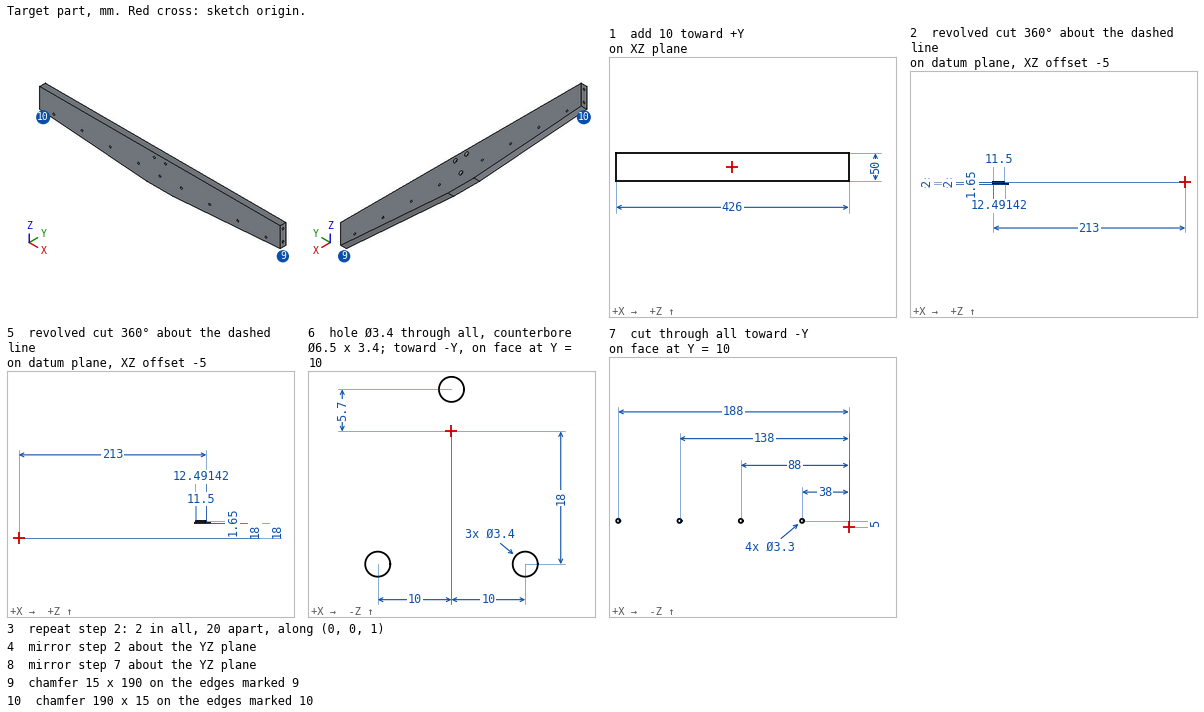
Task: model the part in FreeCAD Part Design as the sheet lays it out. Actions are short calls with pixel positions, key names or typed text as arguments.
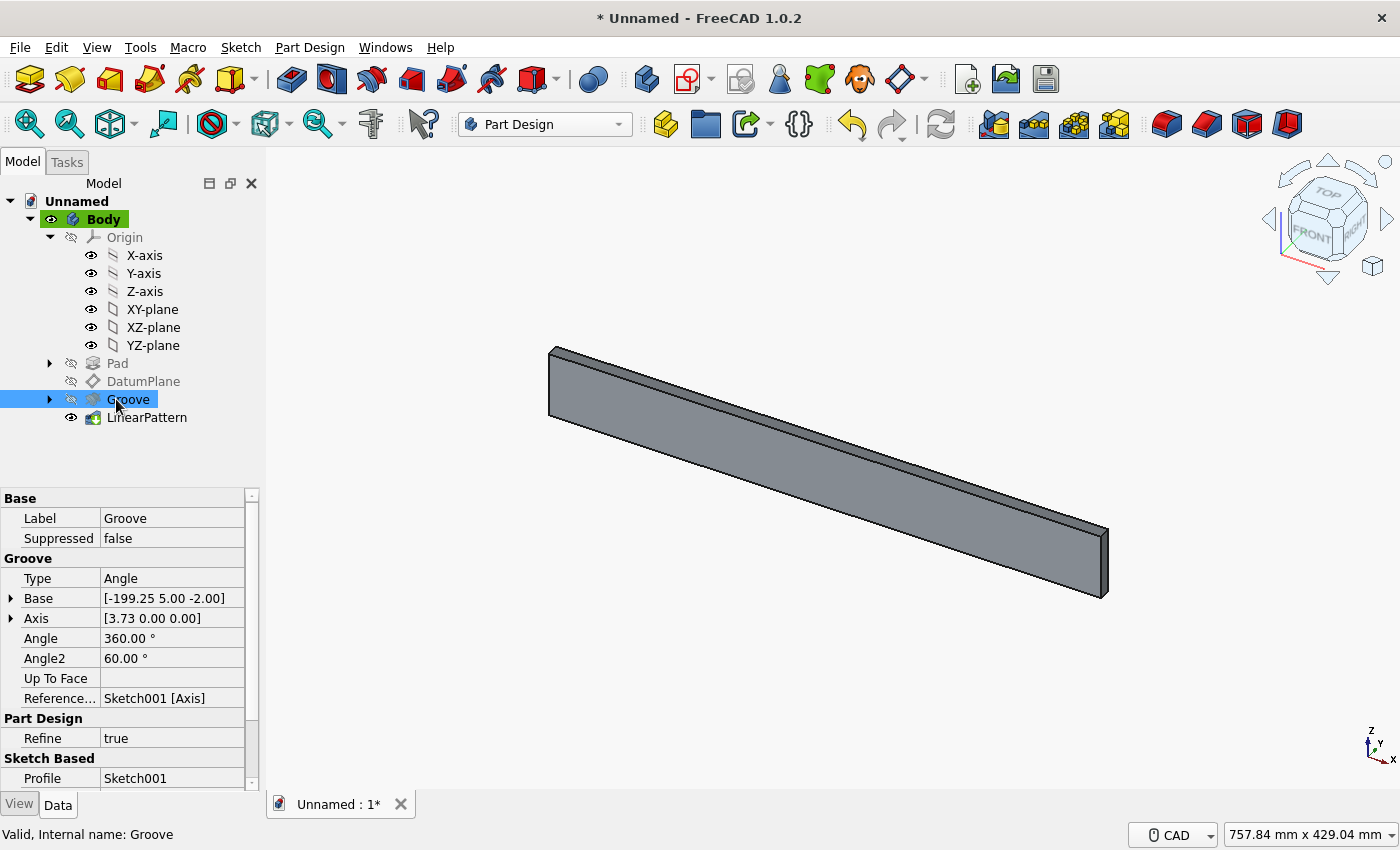
click(994, 124)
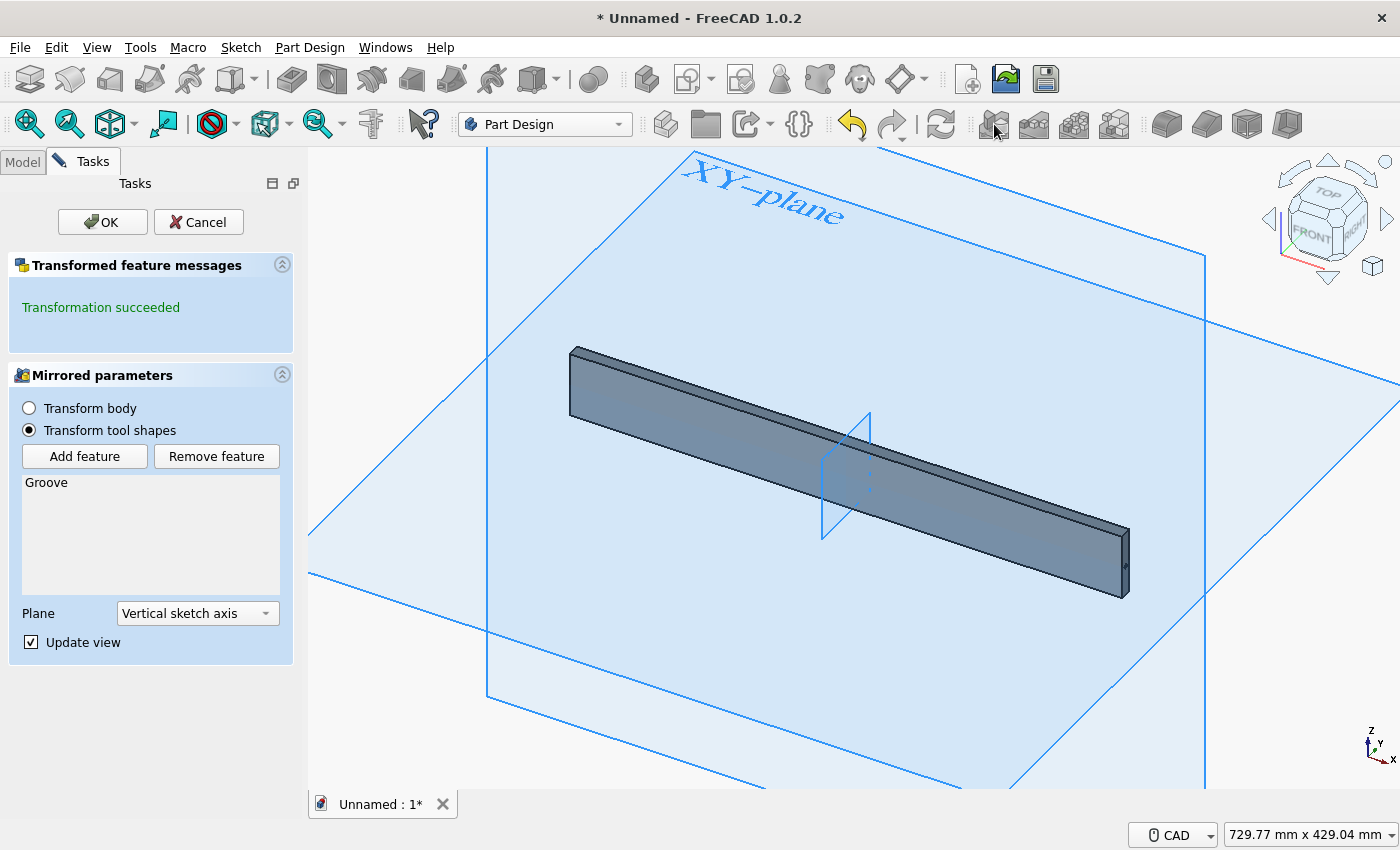
click(198, 614)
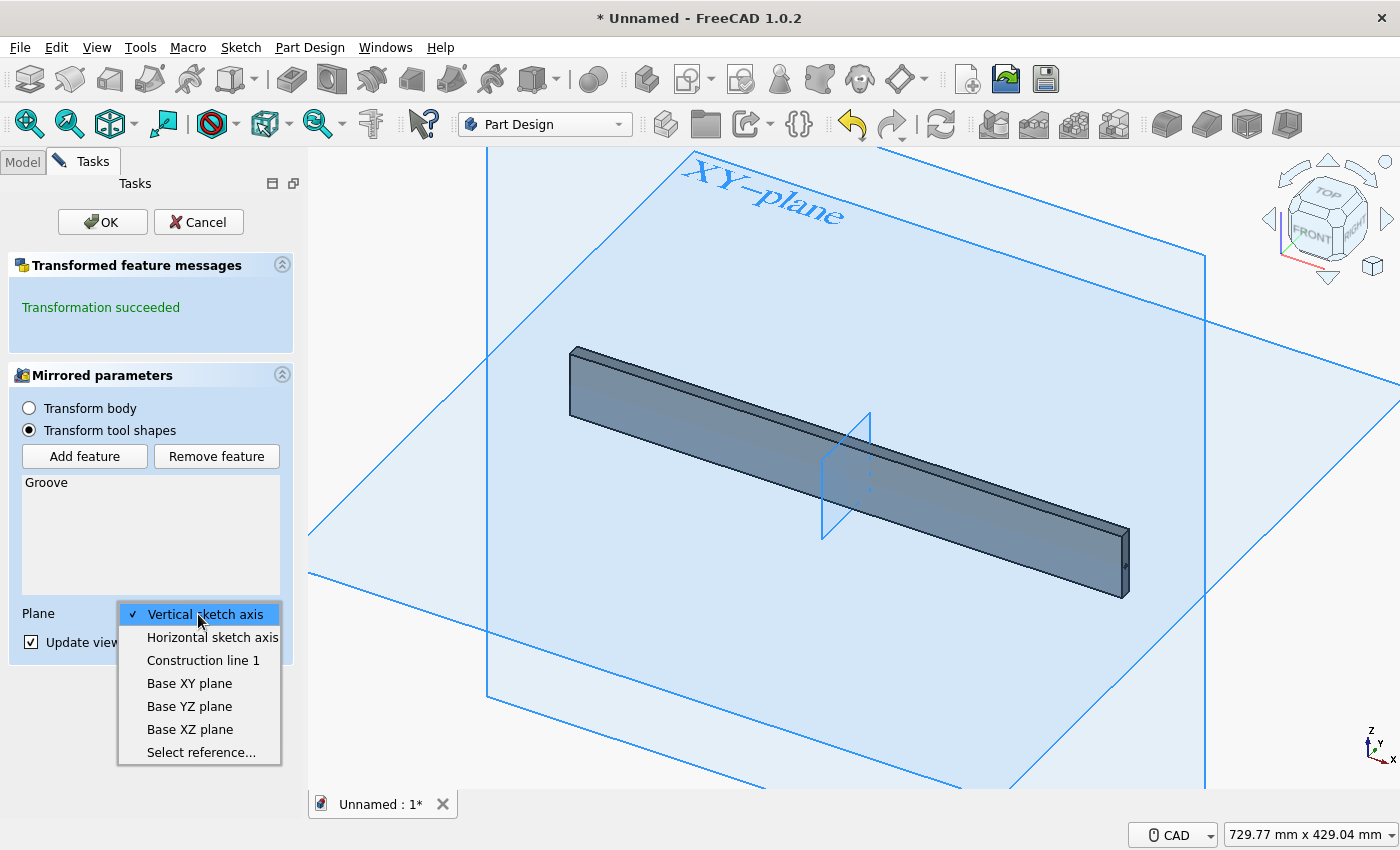
click(198, 706)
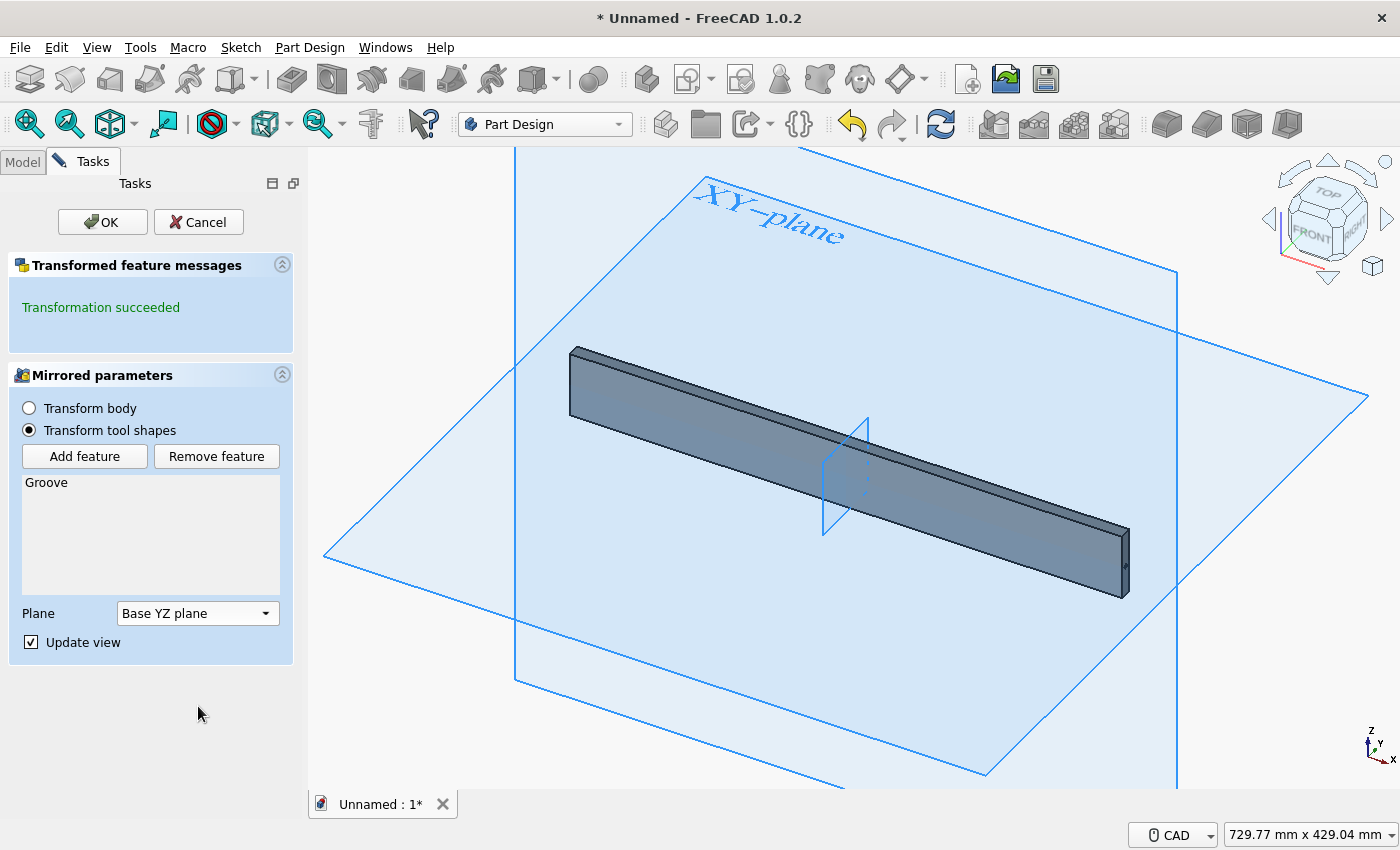
click(103, 222)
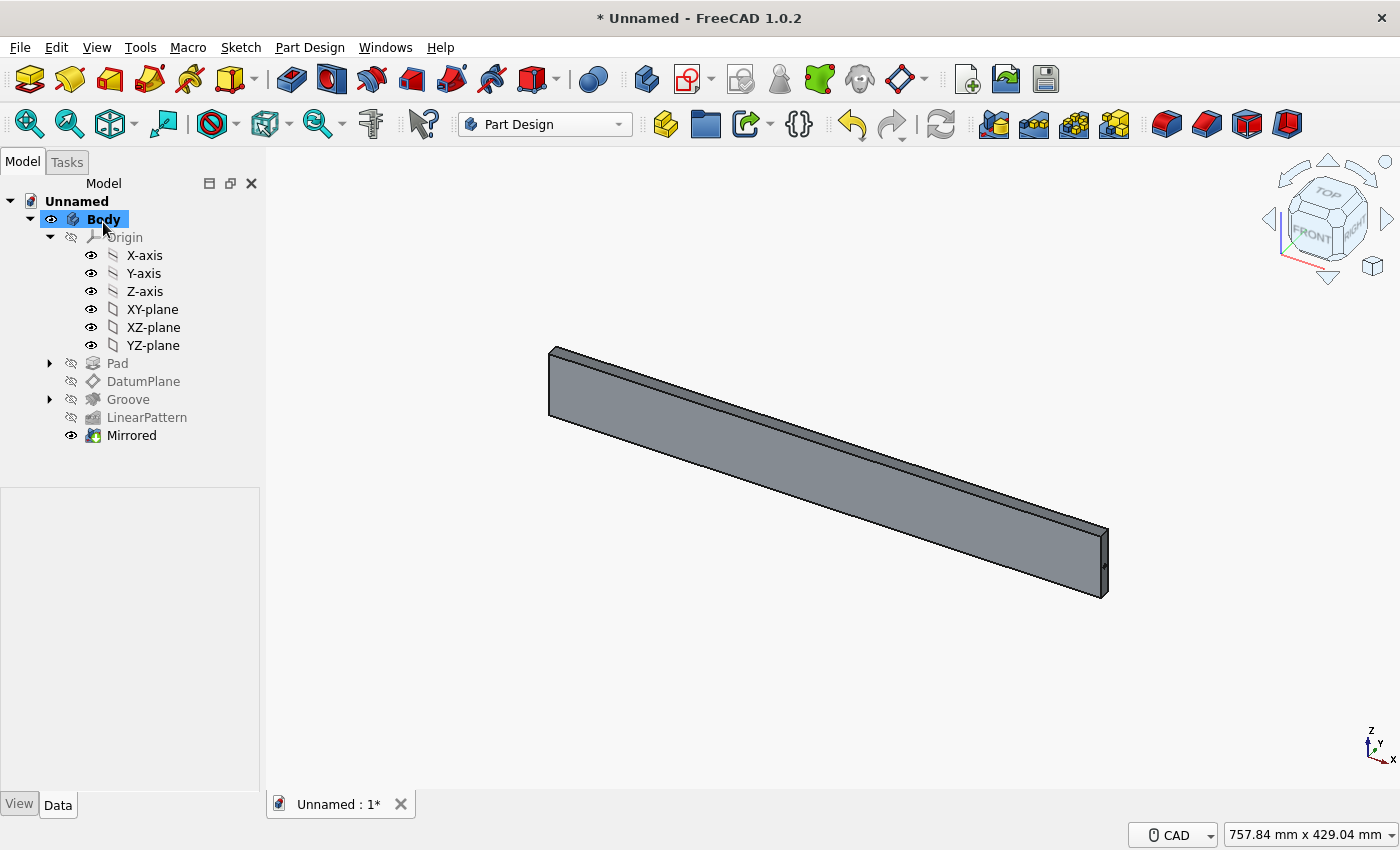
click(136, 327)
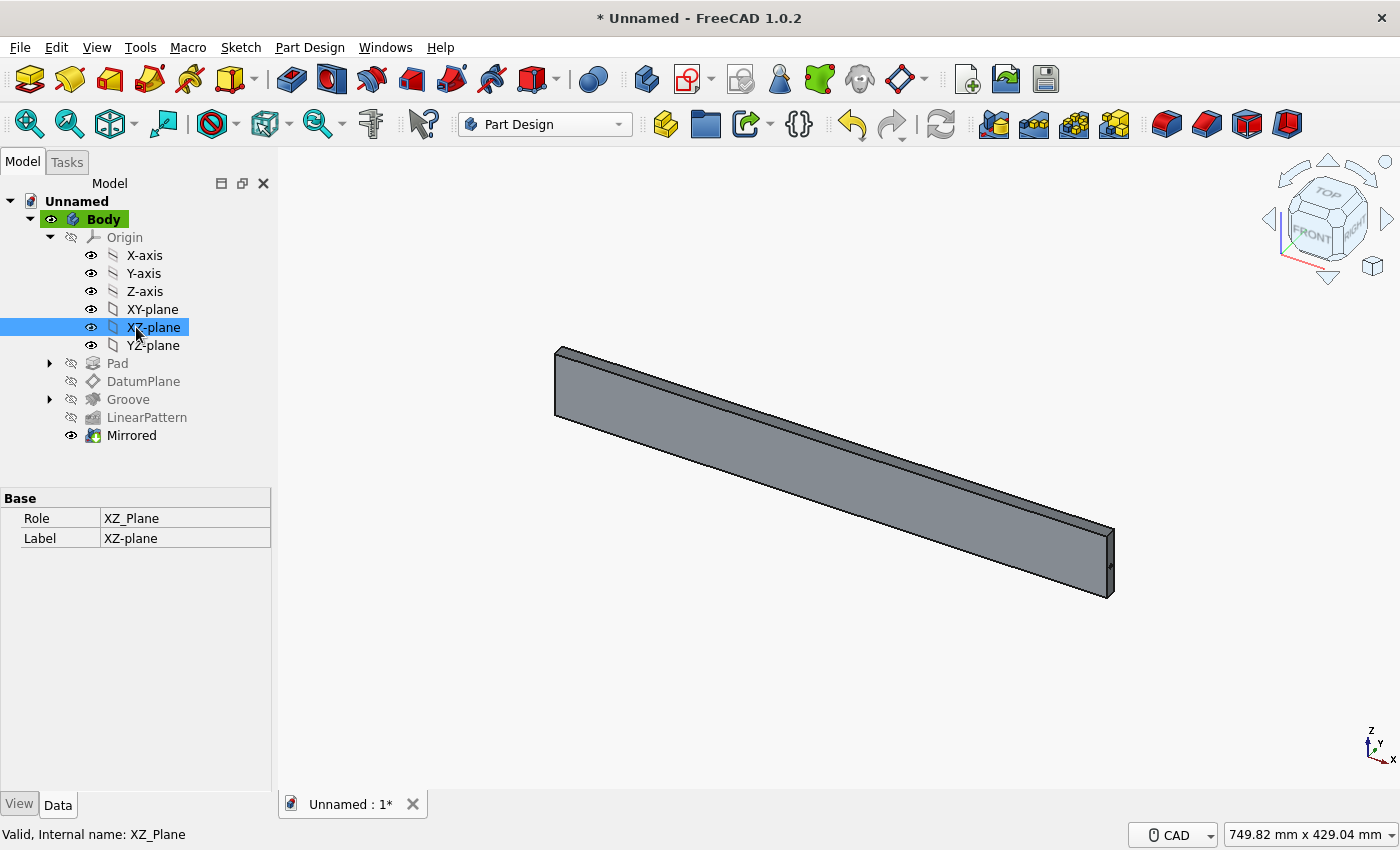
click(900, 80)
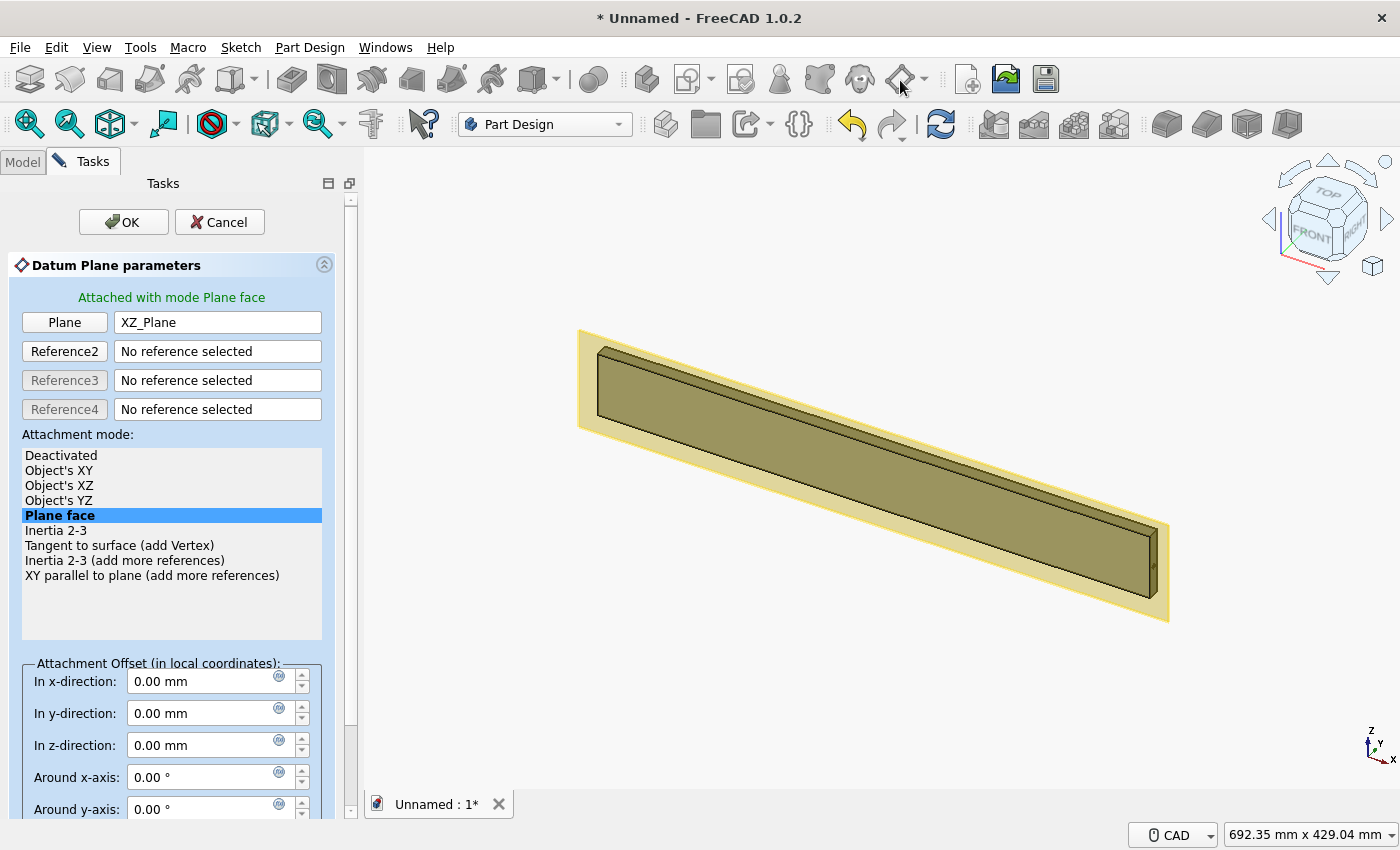
triple_click(210, 745)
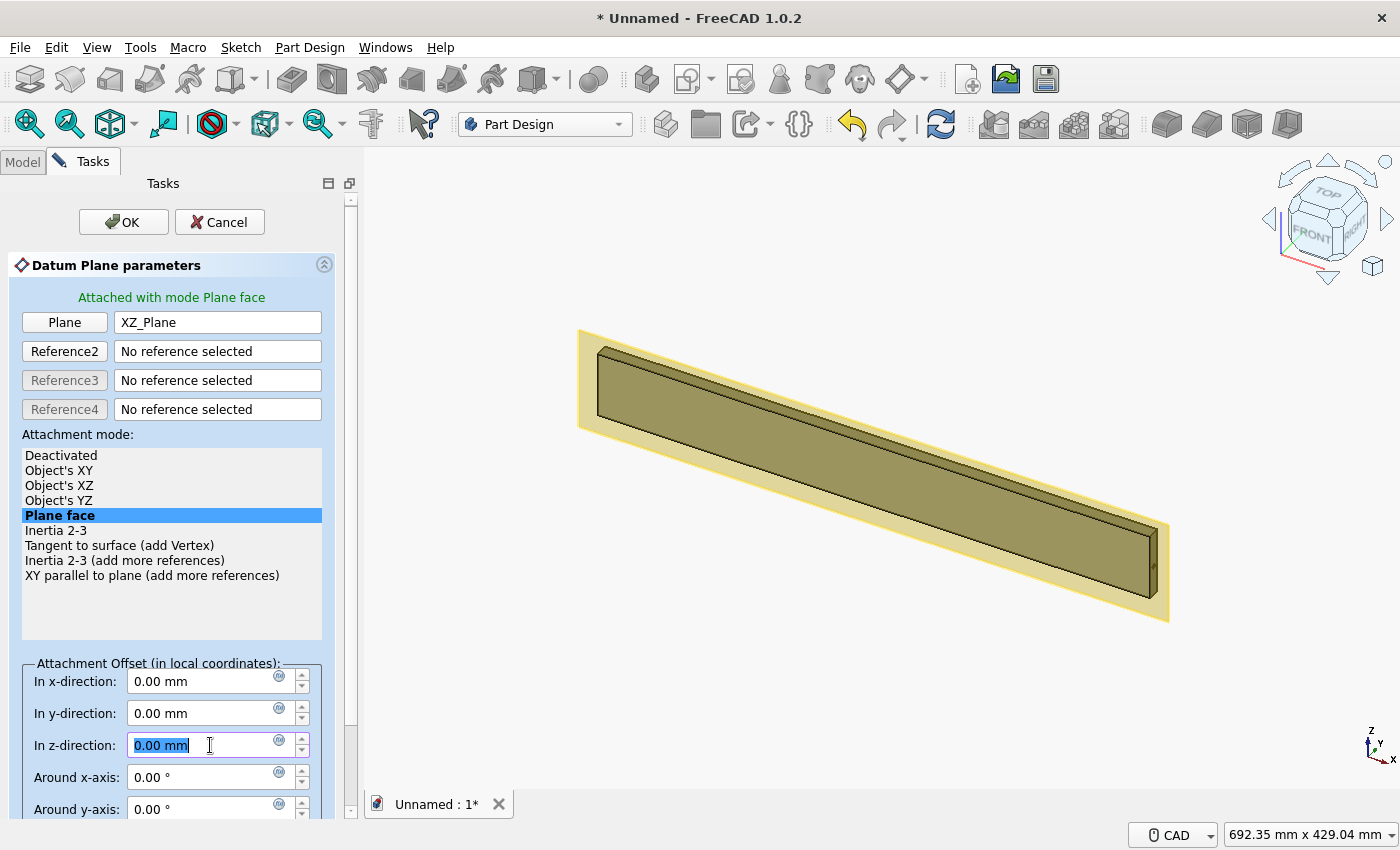
text(-5)
key(Tab)